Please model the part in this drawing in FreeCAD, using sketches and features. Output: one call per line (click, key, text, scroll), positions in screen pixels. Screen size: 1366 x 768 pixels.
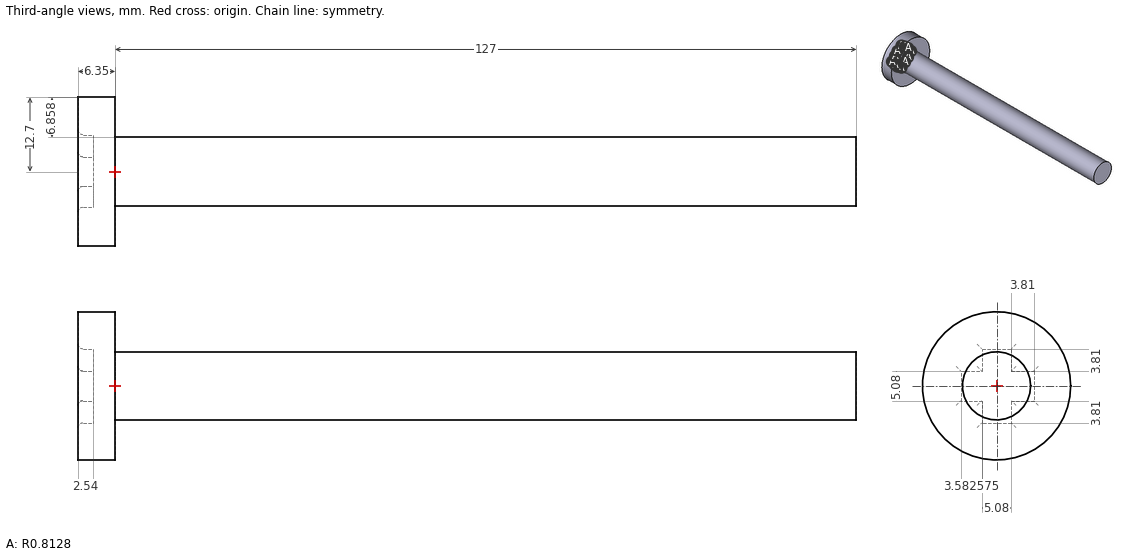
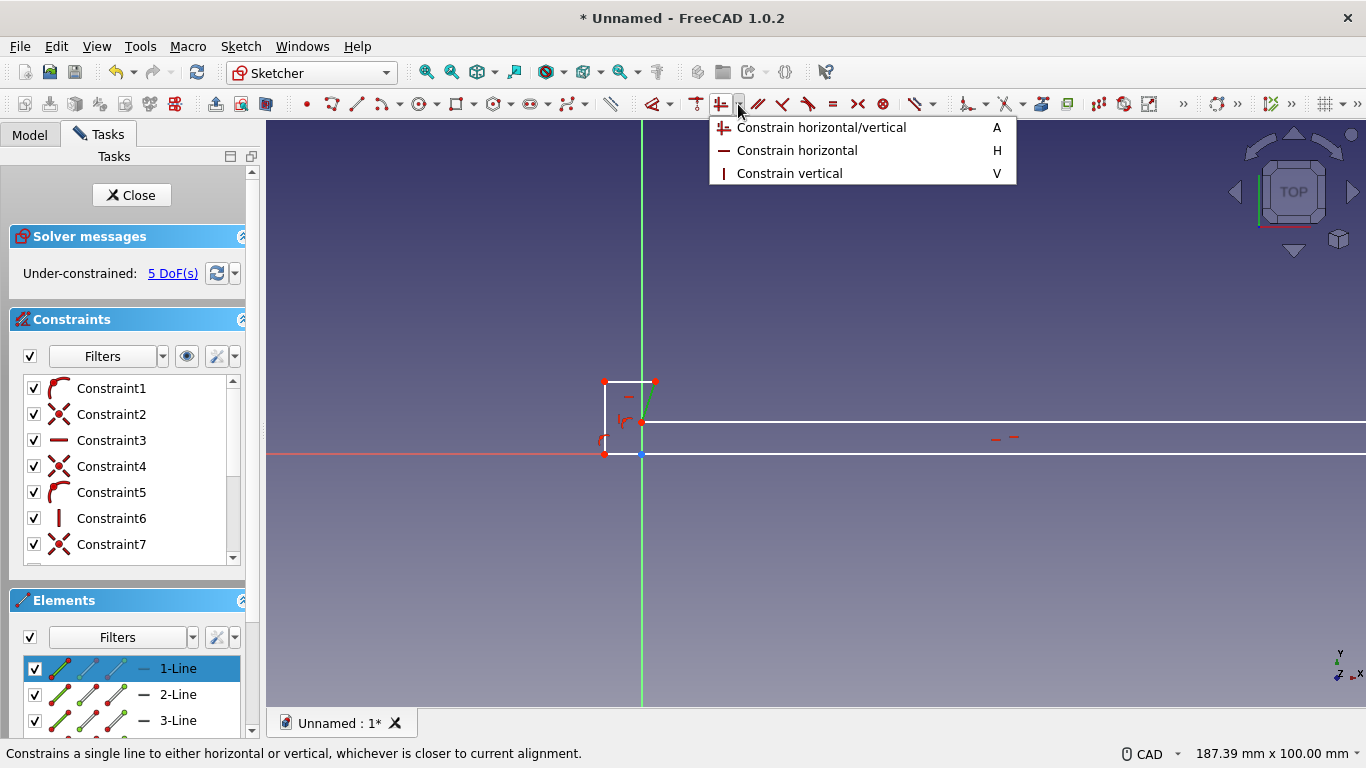
click(863, 174)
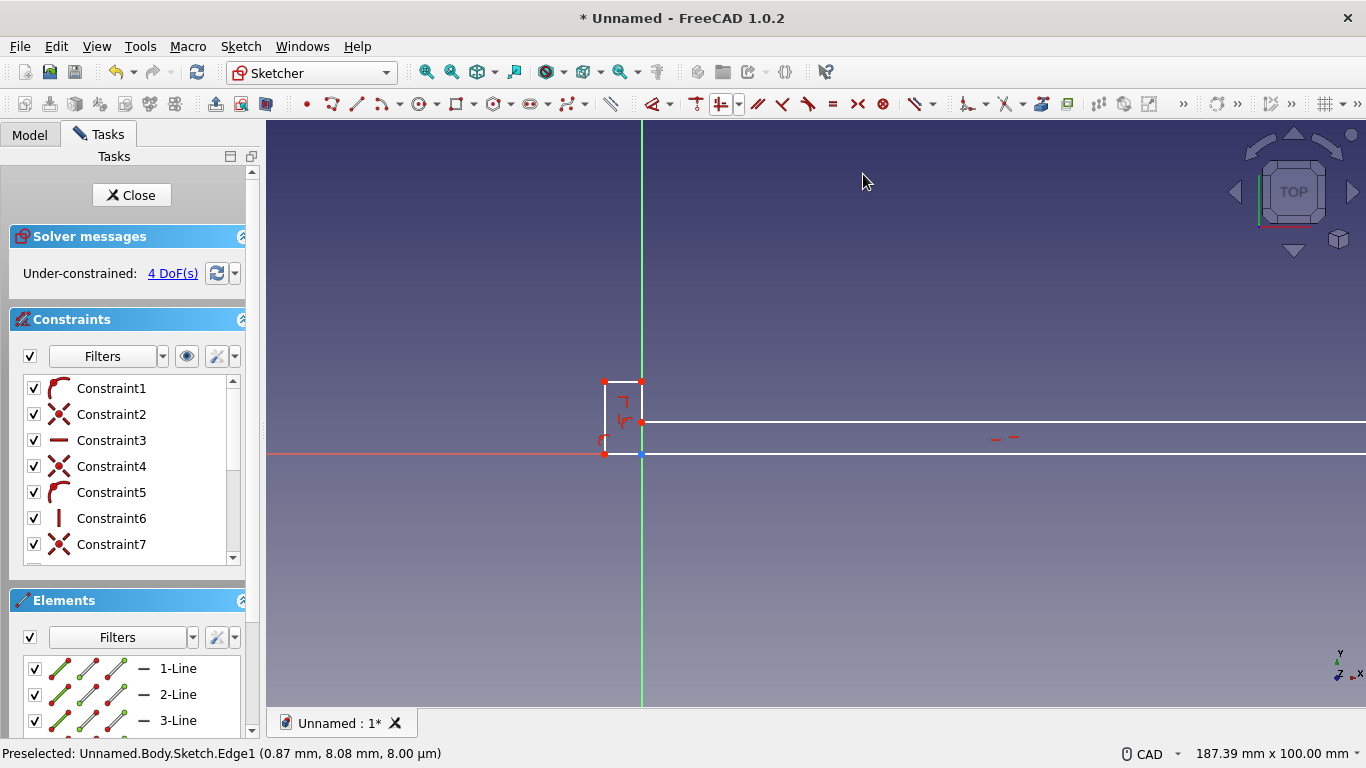
click(652, 104)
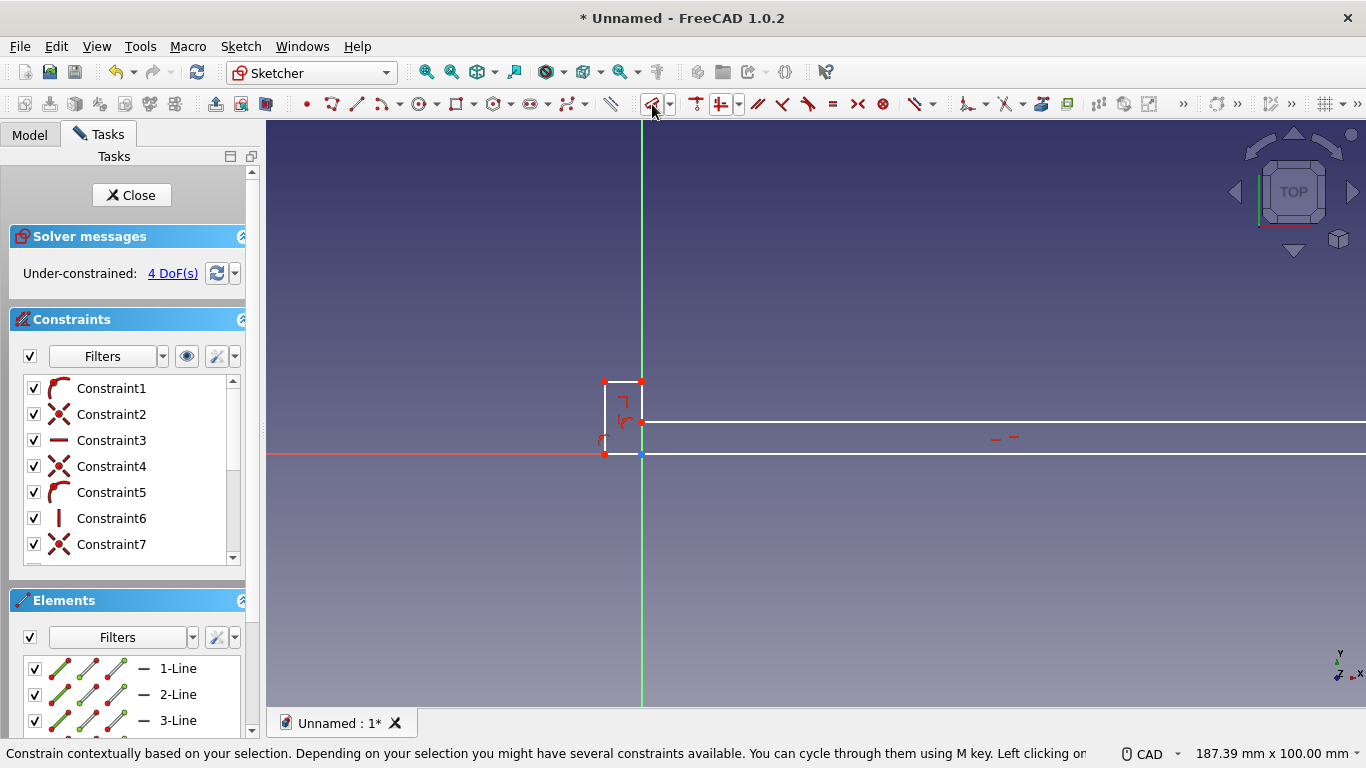
click(1164, 422)
click(921, 388)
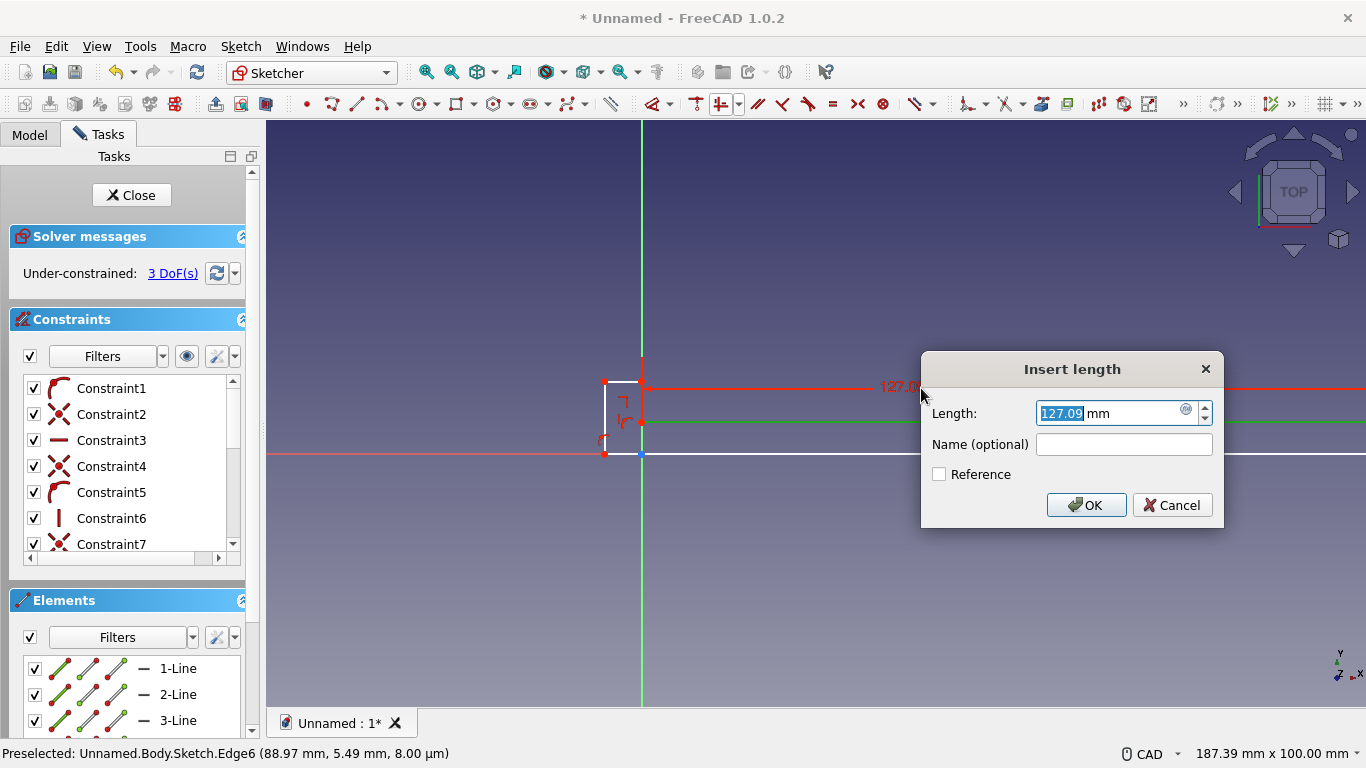
text(127)
key(Return)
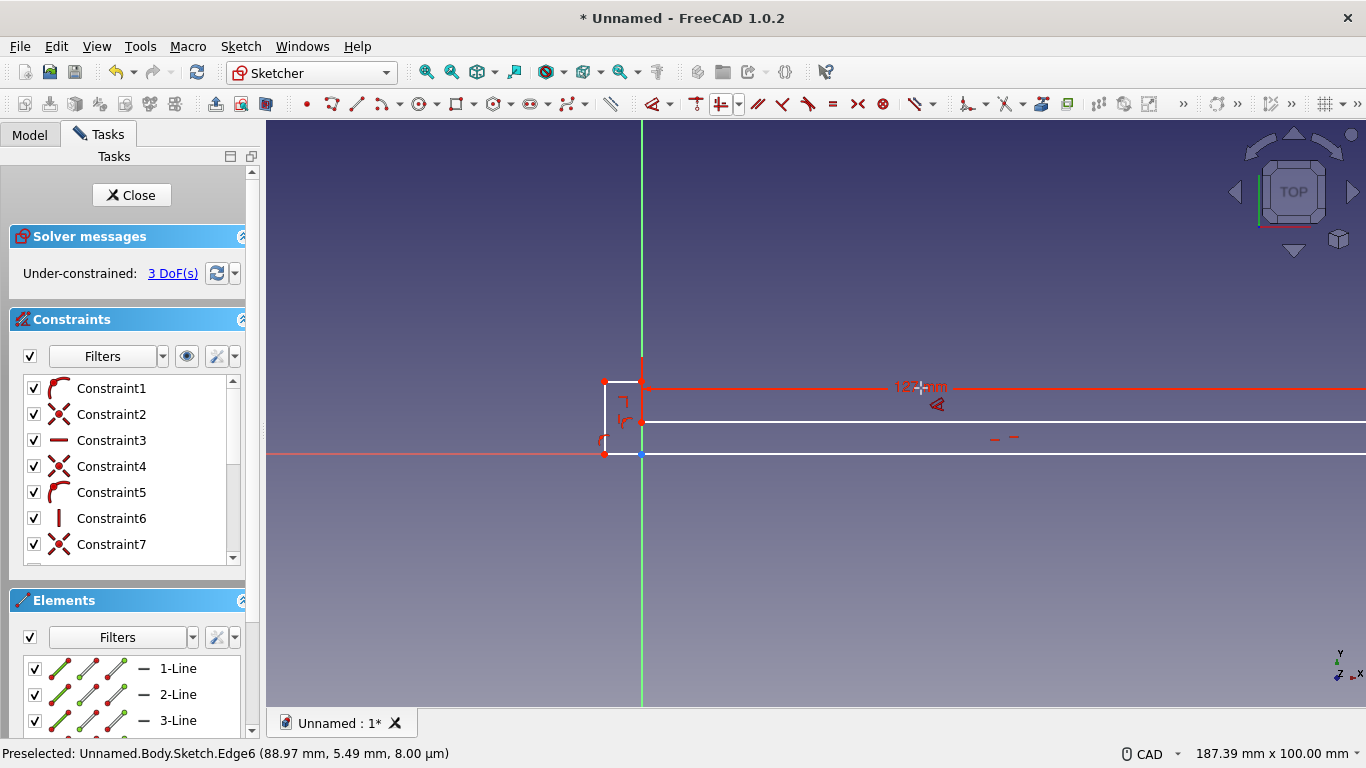
scroll(631, 382, up, 2)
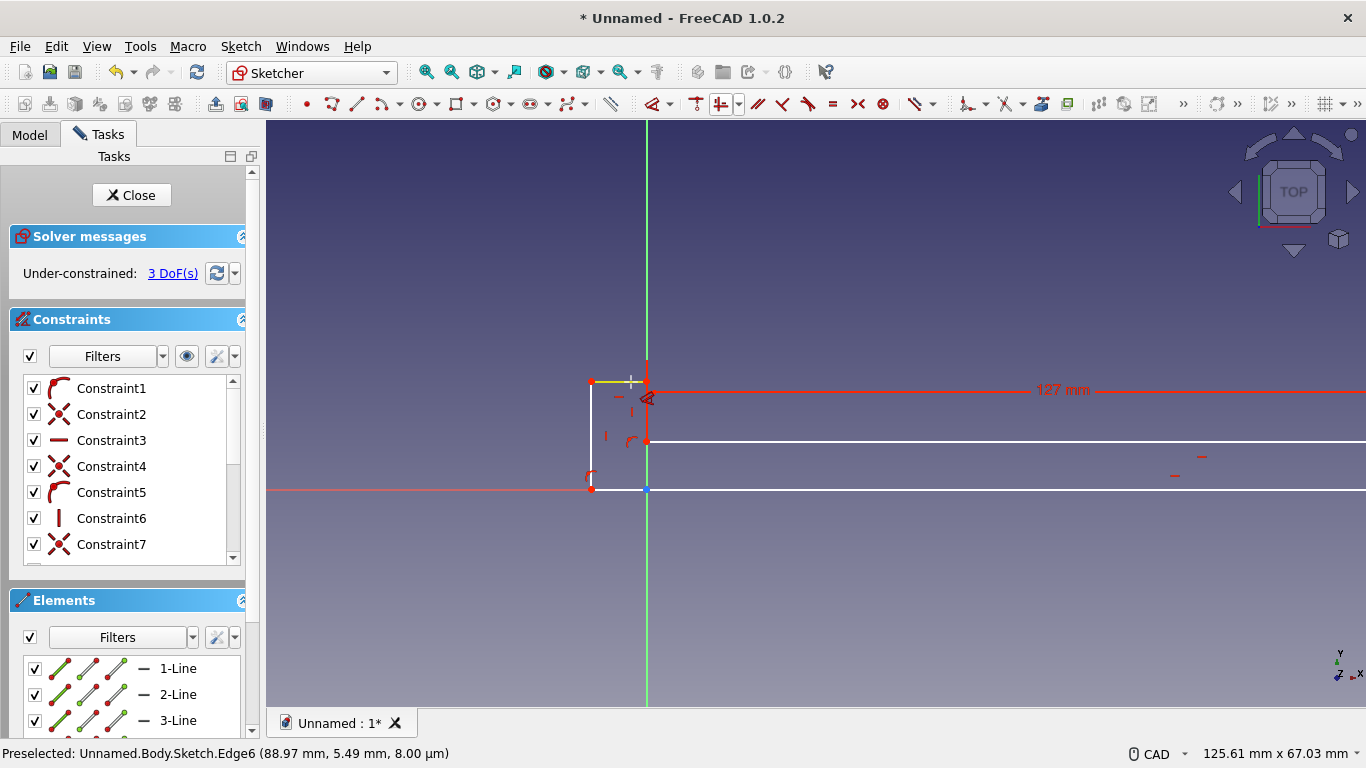
click(630, 382)
click(619, 348)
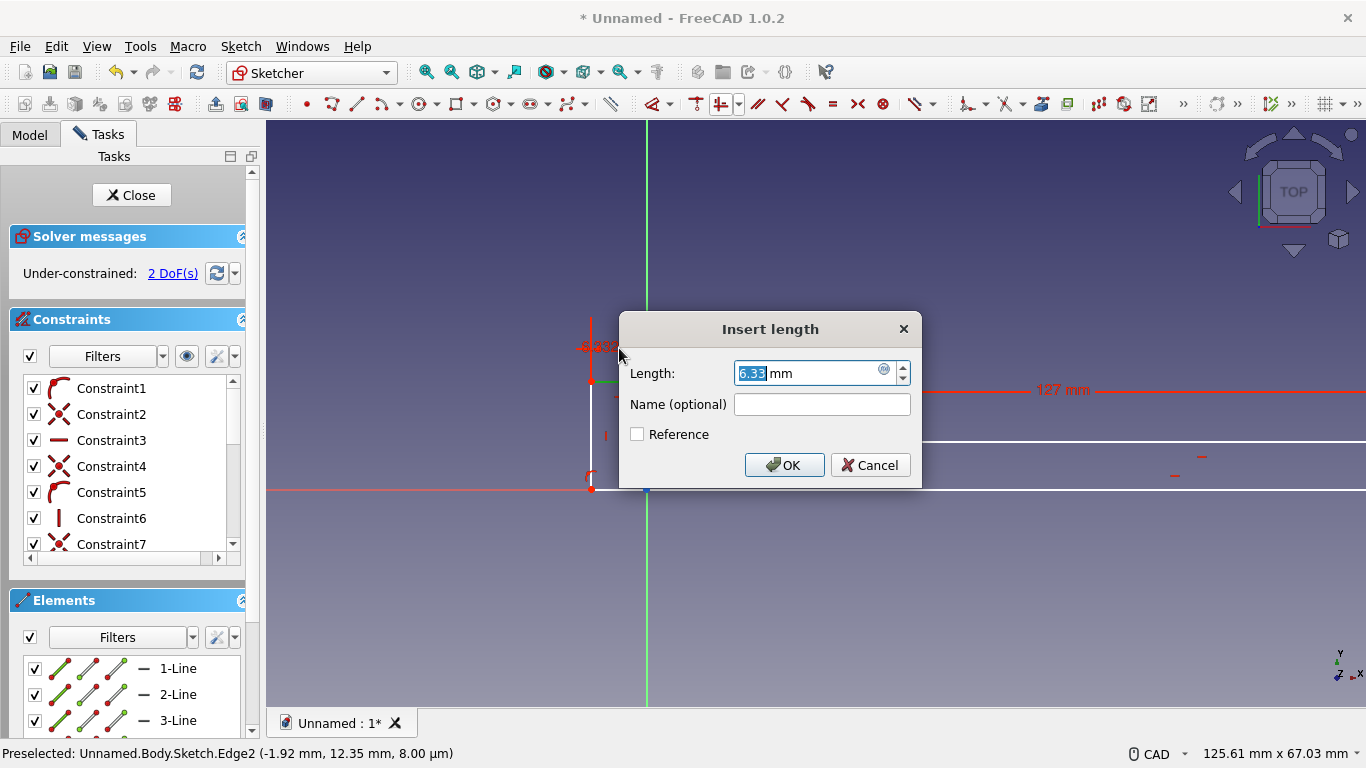
text(6.35)
key(Return)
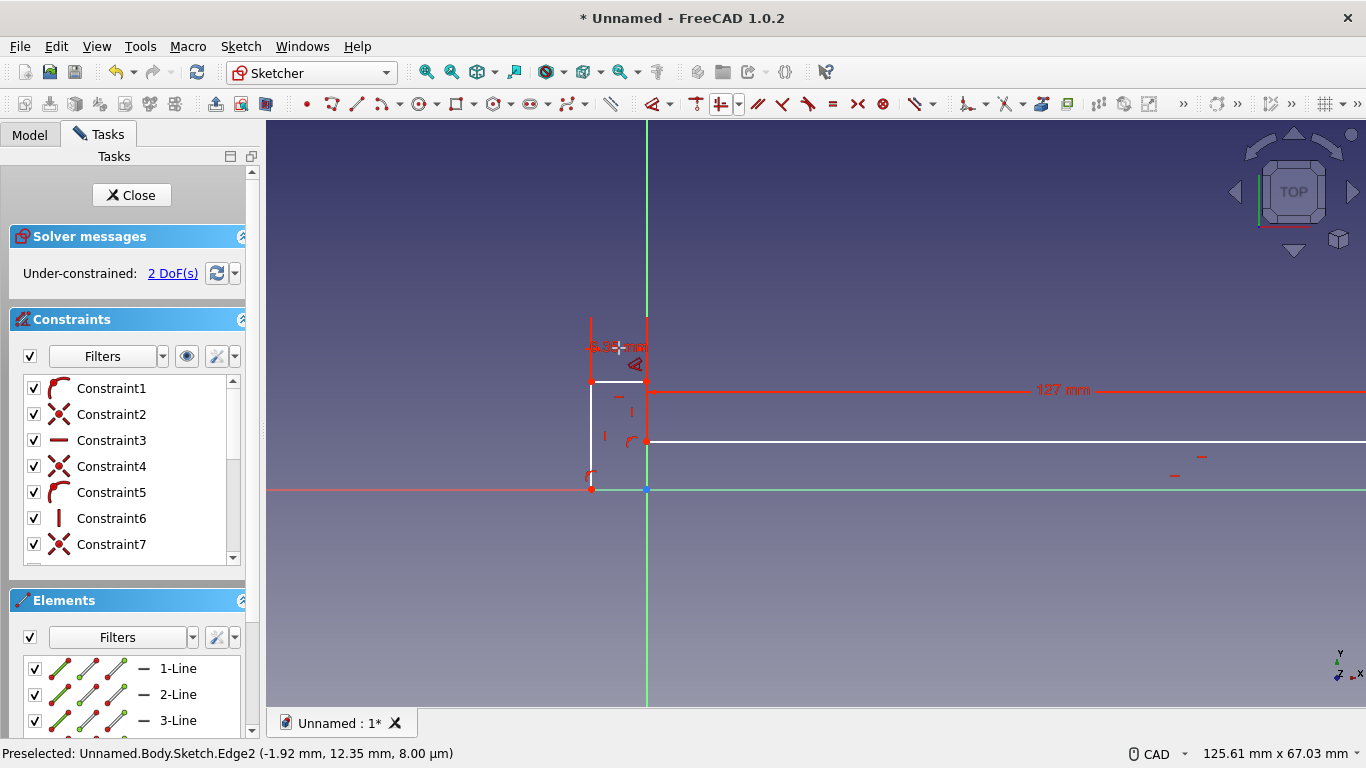
click(591, 414)
click(557, 436)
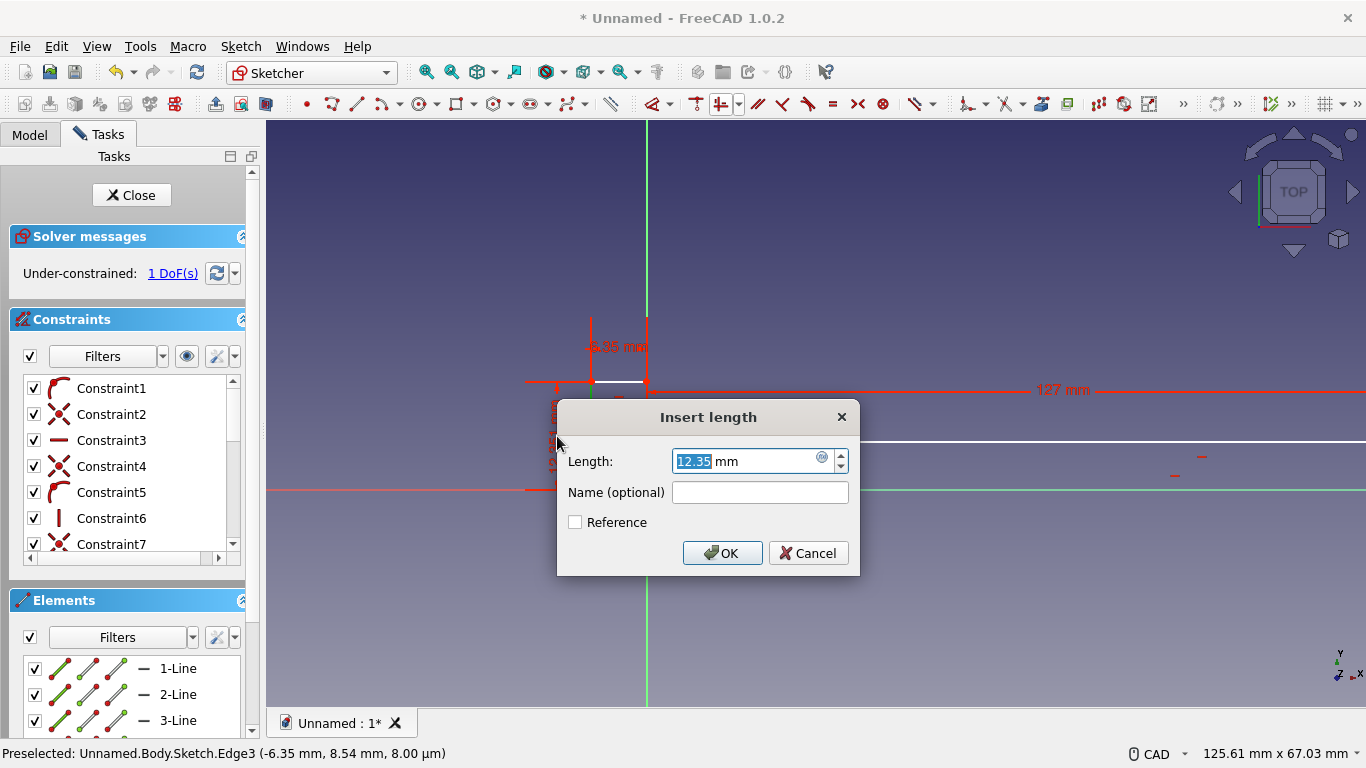
text(12.7)
key(Return)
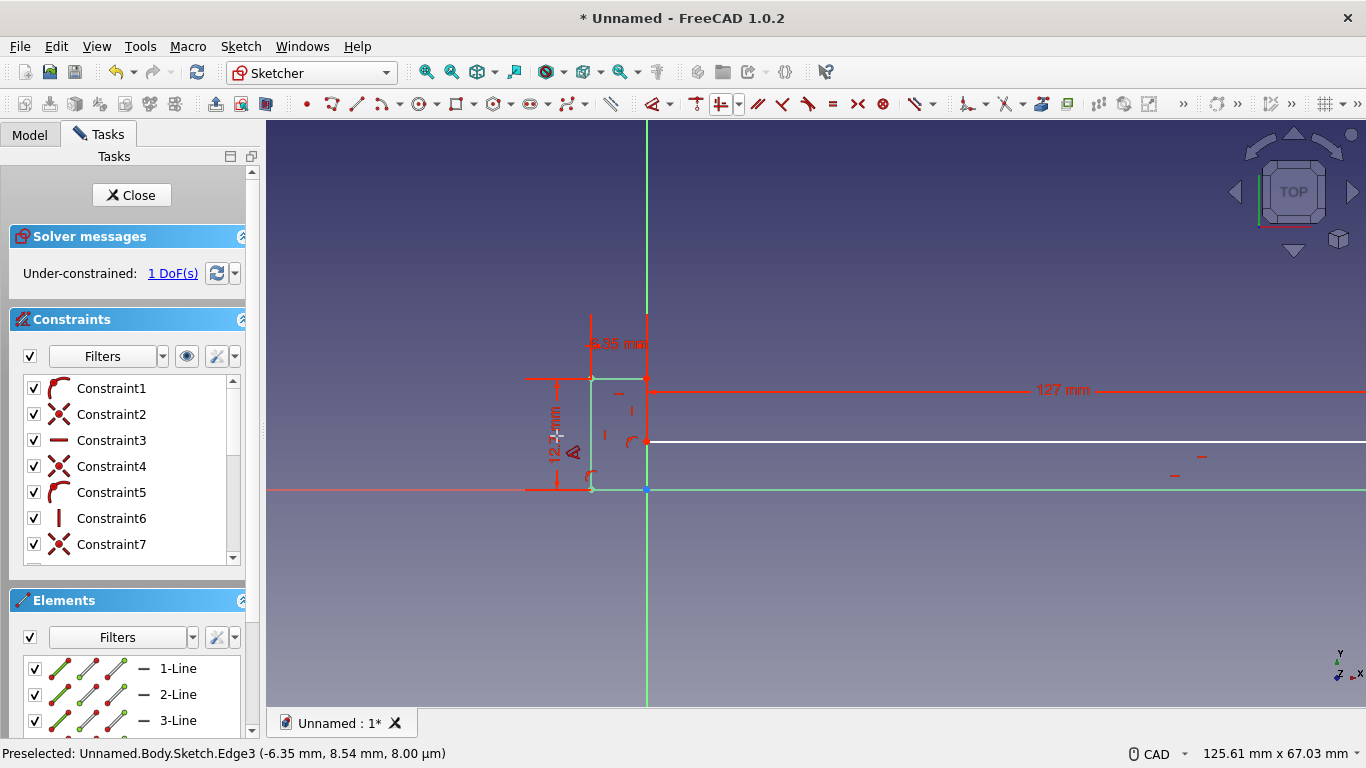
click(647, 423)
click(613, 410)